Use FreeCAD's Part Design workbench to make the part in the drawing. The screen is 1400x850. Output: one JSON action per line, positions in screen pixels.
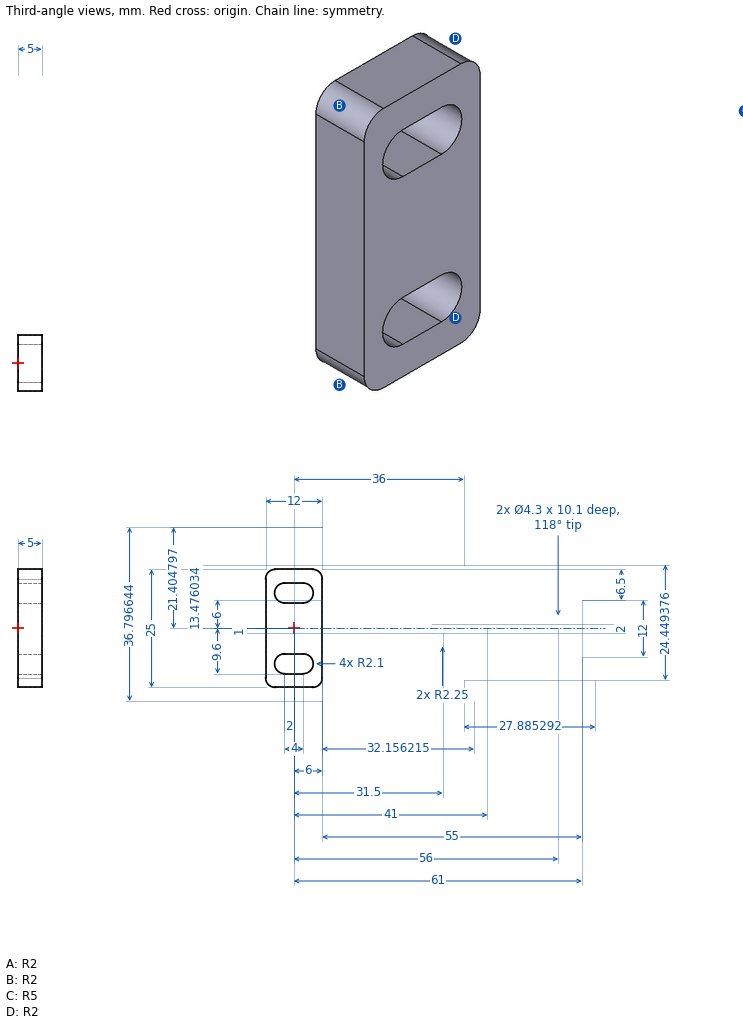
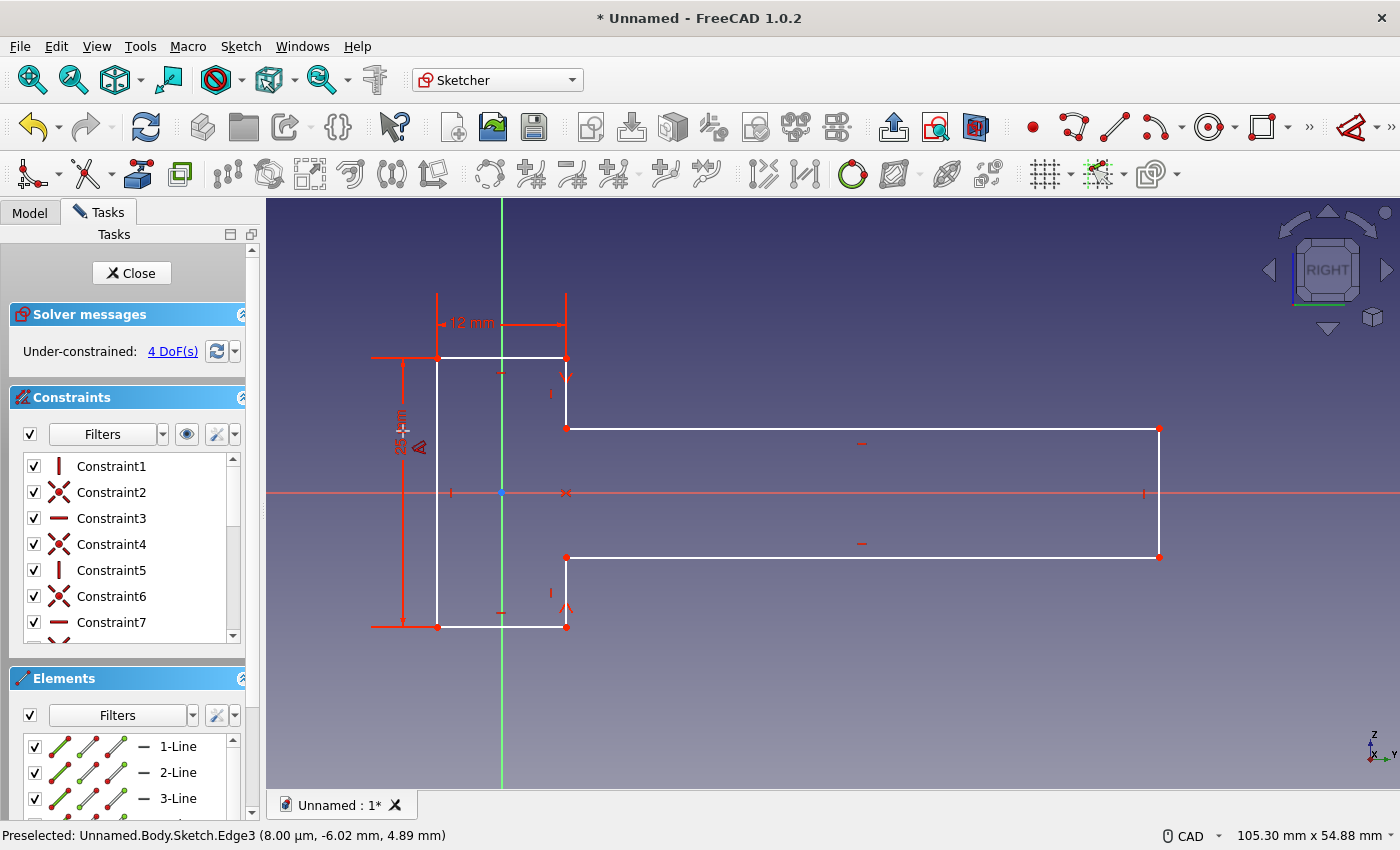
{"action": "left_click", "coordinate": [744, 558]}
{"action": "left_click", "coordinate": [863, 592]}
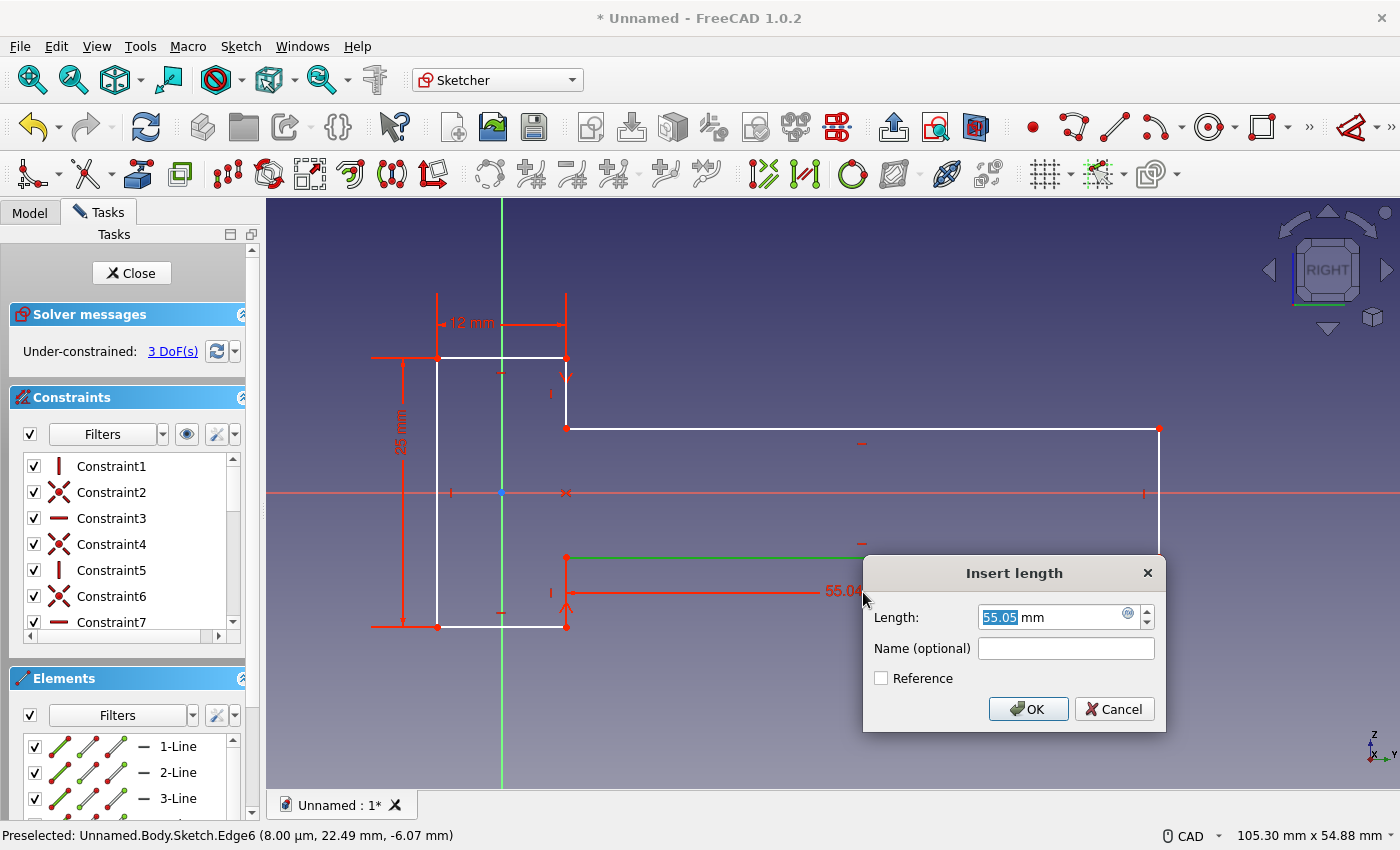
{"action": "type", "text": "55"}
{"action": "key", "text": "Return"}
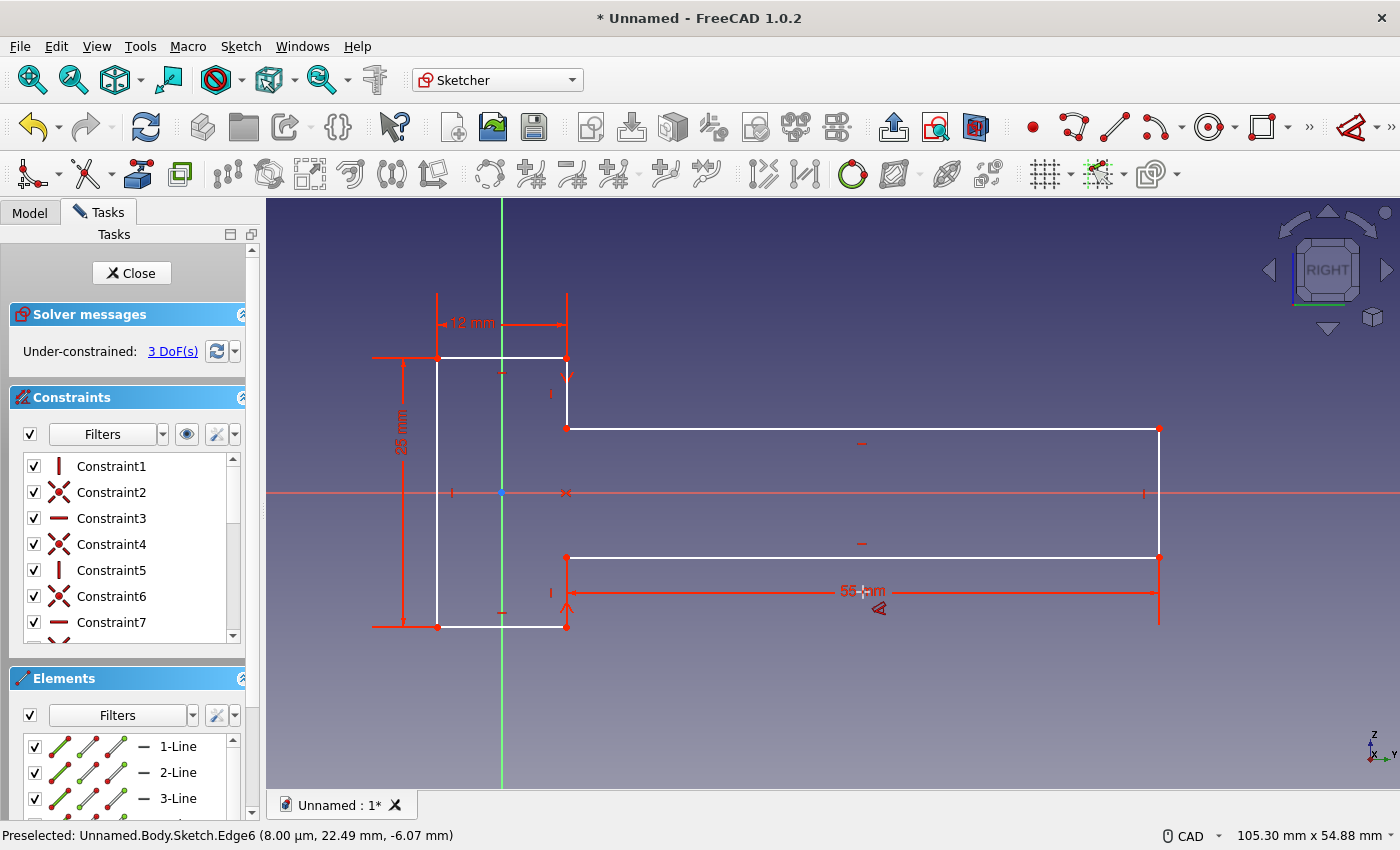
{"action": "left_click", "coordinate": [1159, 519]}
{"action": "left_click", "coordinate": [1193, 464]}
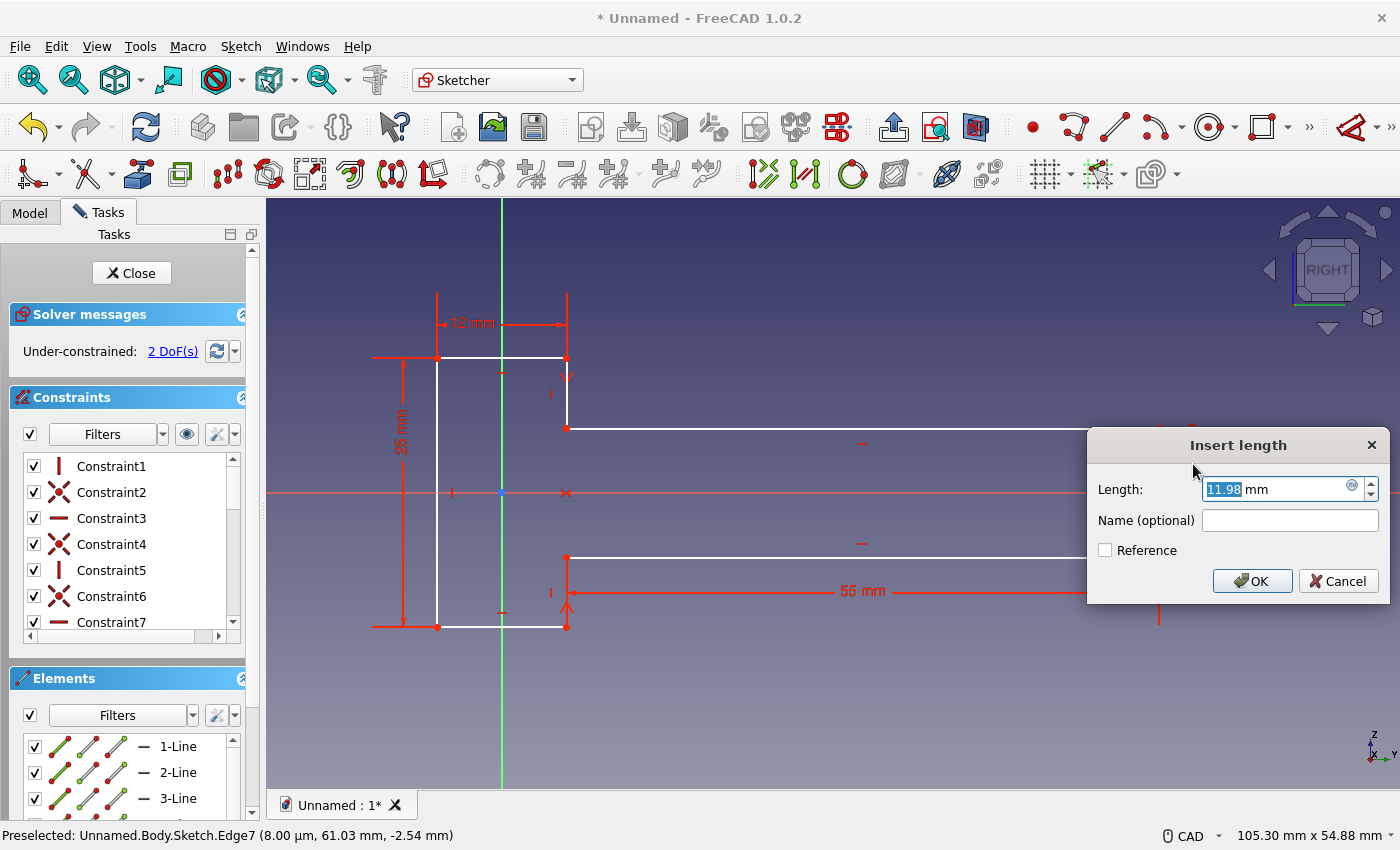
{"action": "type", "text": "12"}
{"action": "key", "text": "Return"}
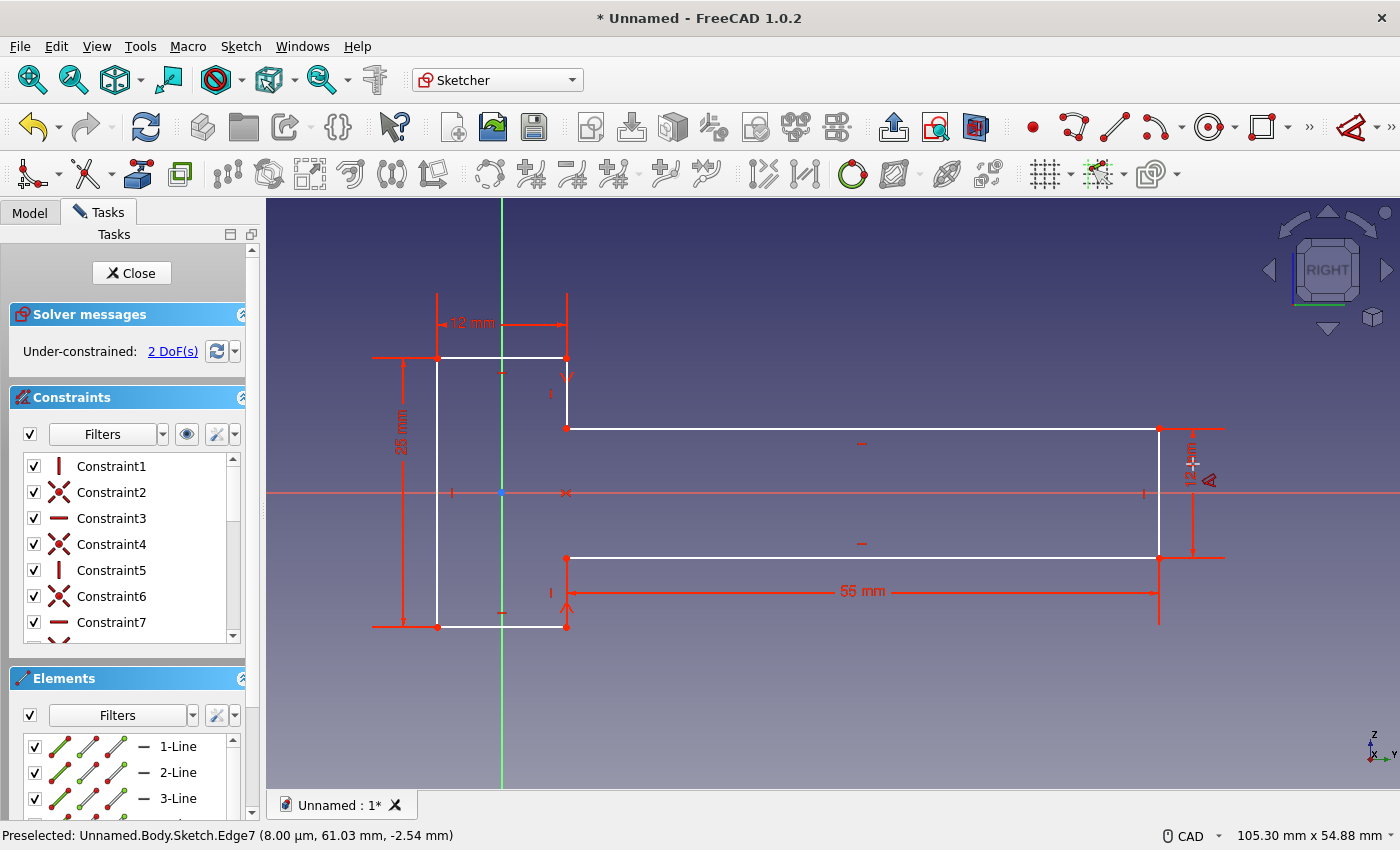
{"action": "left_click", "coordinate": [567, 429]}
{"action": "left_click", "coordinate": [534, 395]}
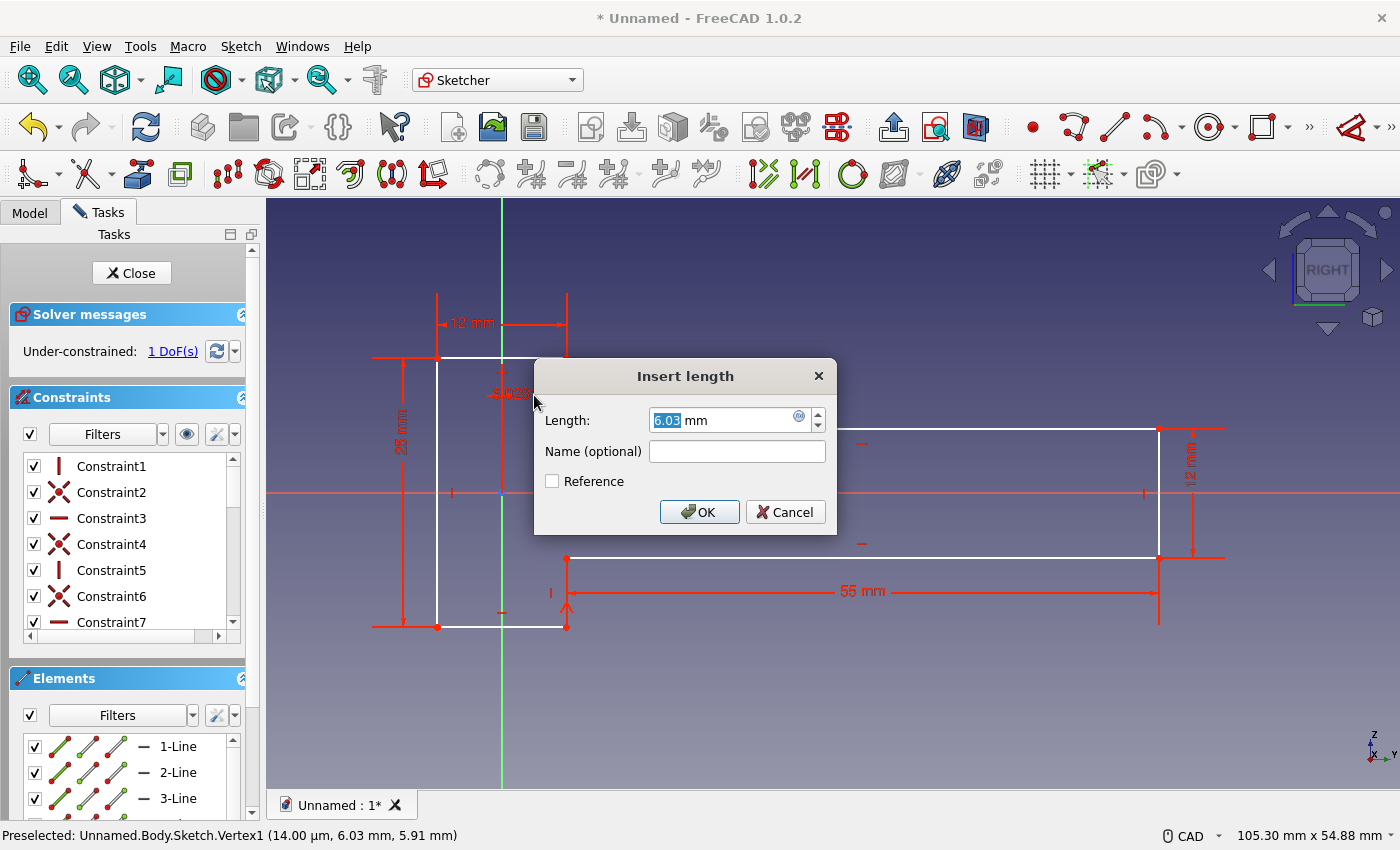
{"action": "type", "text": "6"}
{"action": "key", "text": "Return"}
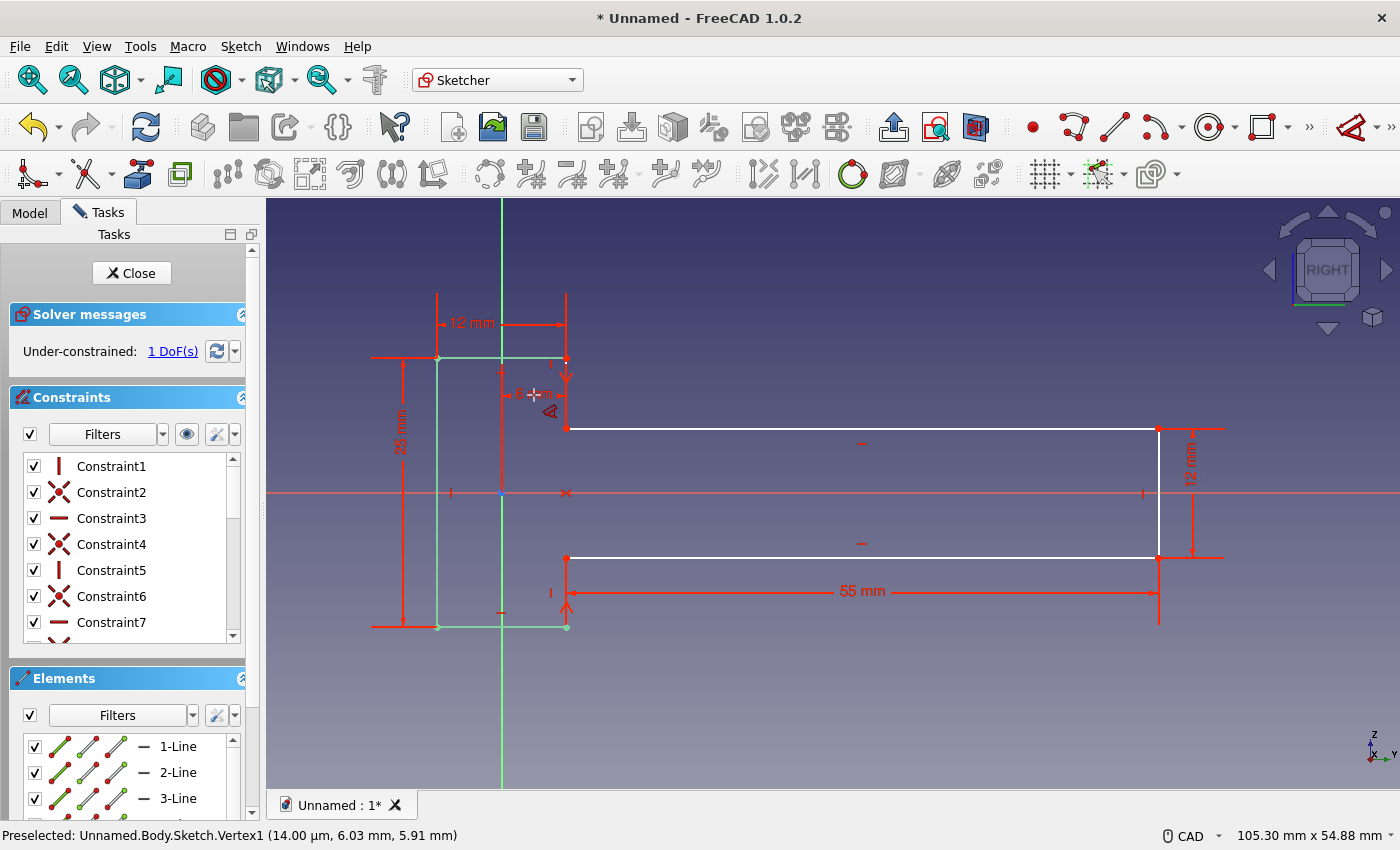
{"action": "left_click", "coordinate": [566, 429]}
{"action": "left_click", "coordinate": [468, 461]}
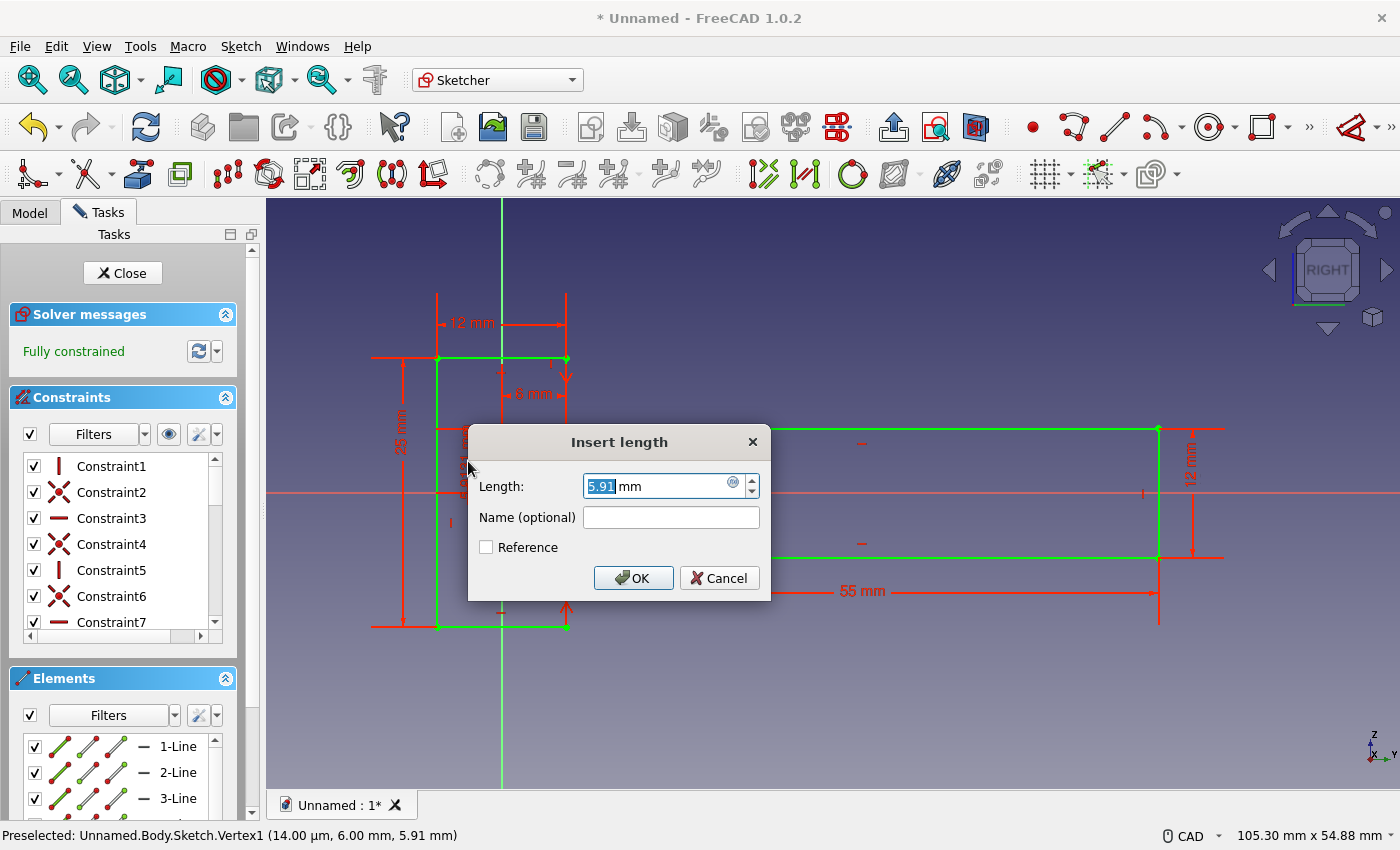
{"action": "type", "text": "6"}
{"action": "key", "text": "Return"}
{"action": "key", "text": "Escape"}